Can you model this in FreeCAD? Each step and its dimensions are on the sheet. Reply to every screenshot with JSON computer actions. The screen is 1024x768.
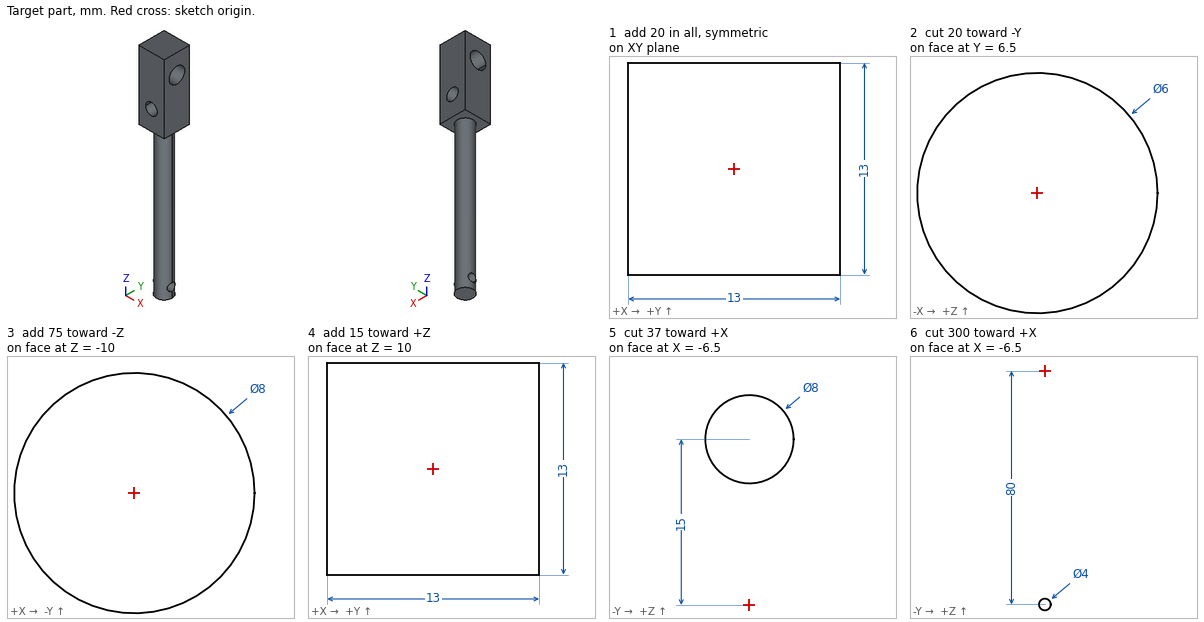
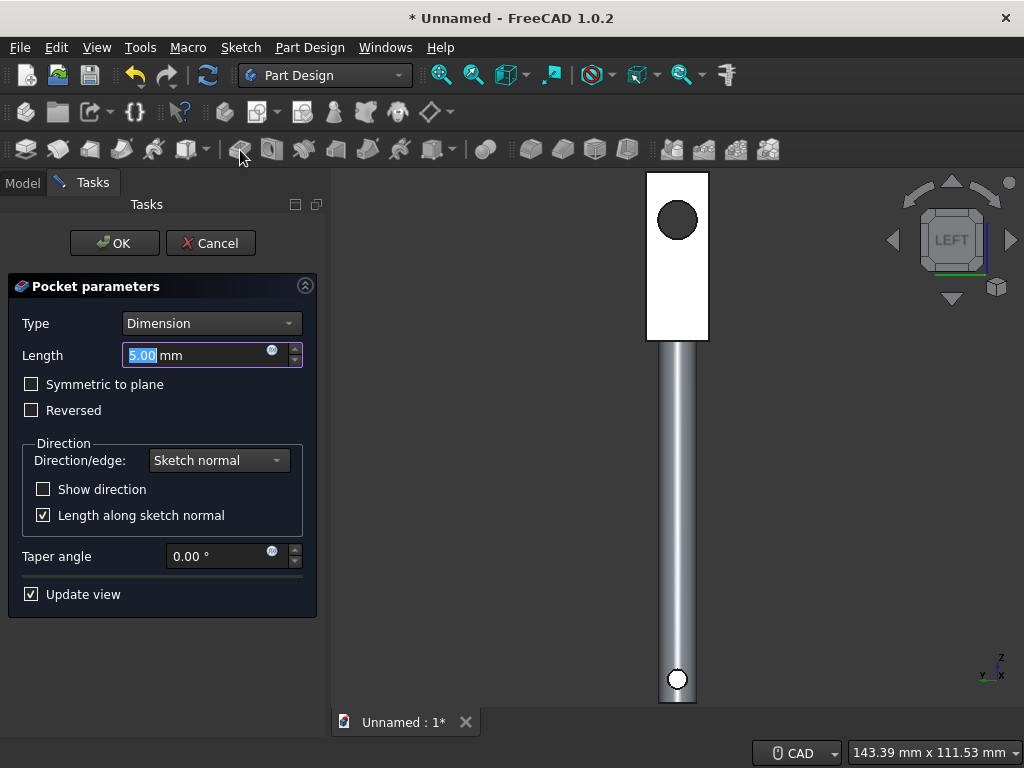
{"action": "type", "text": "300"}
{"action": "key", "text": "Tab"}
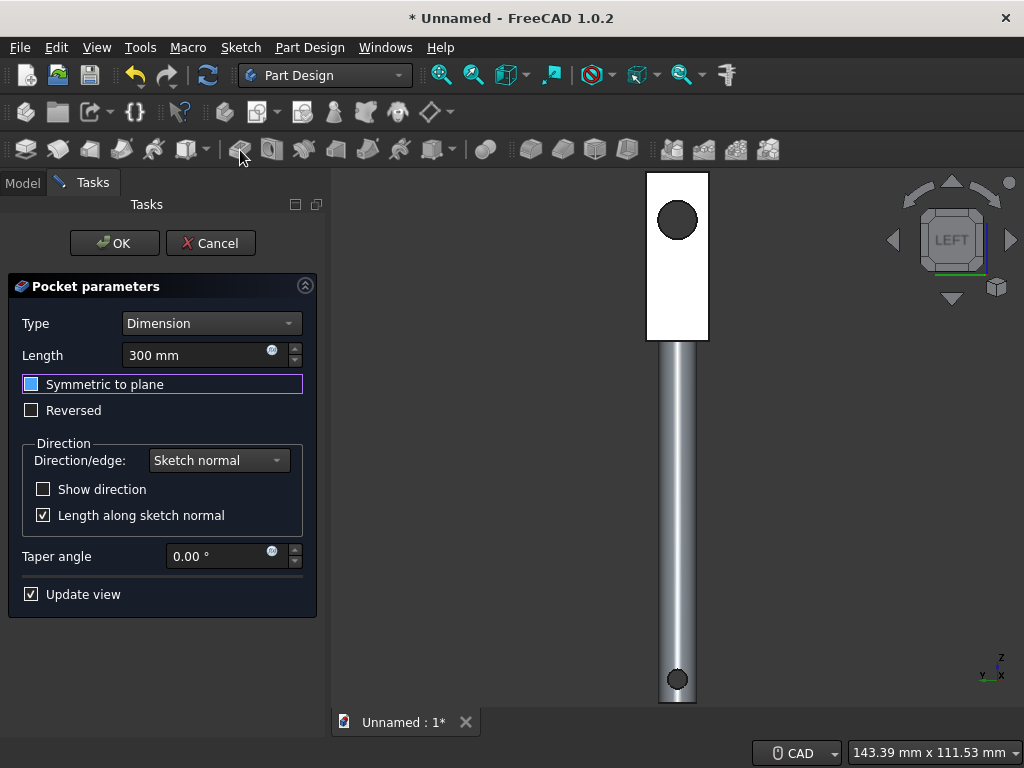
{"action": "left_click", "coordinate": [115, 243]}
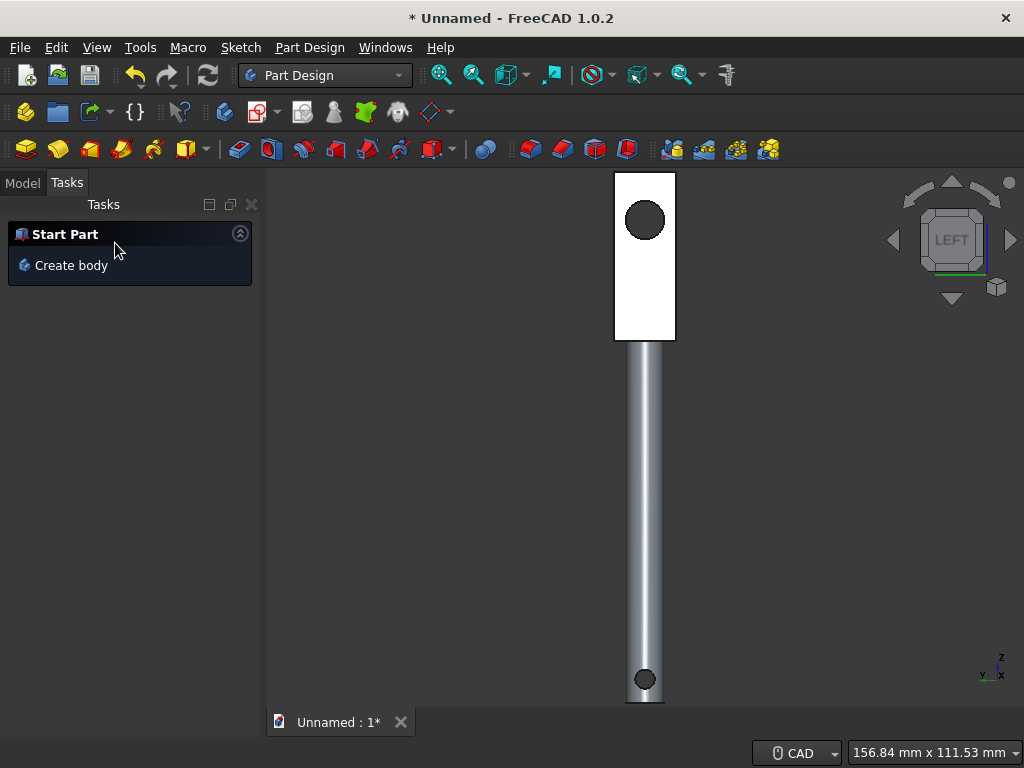
{"action": "key", "text": "0"}